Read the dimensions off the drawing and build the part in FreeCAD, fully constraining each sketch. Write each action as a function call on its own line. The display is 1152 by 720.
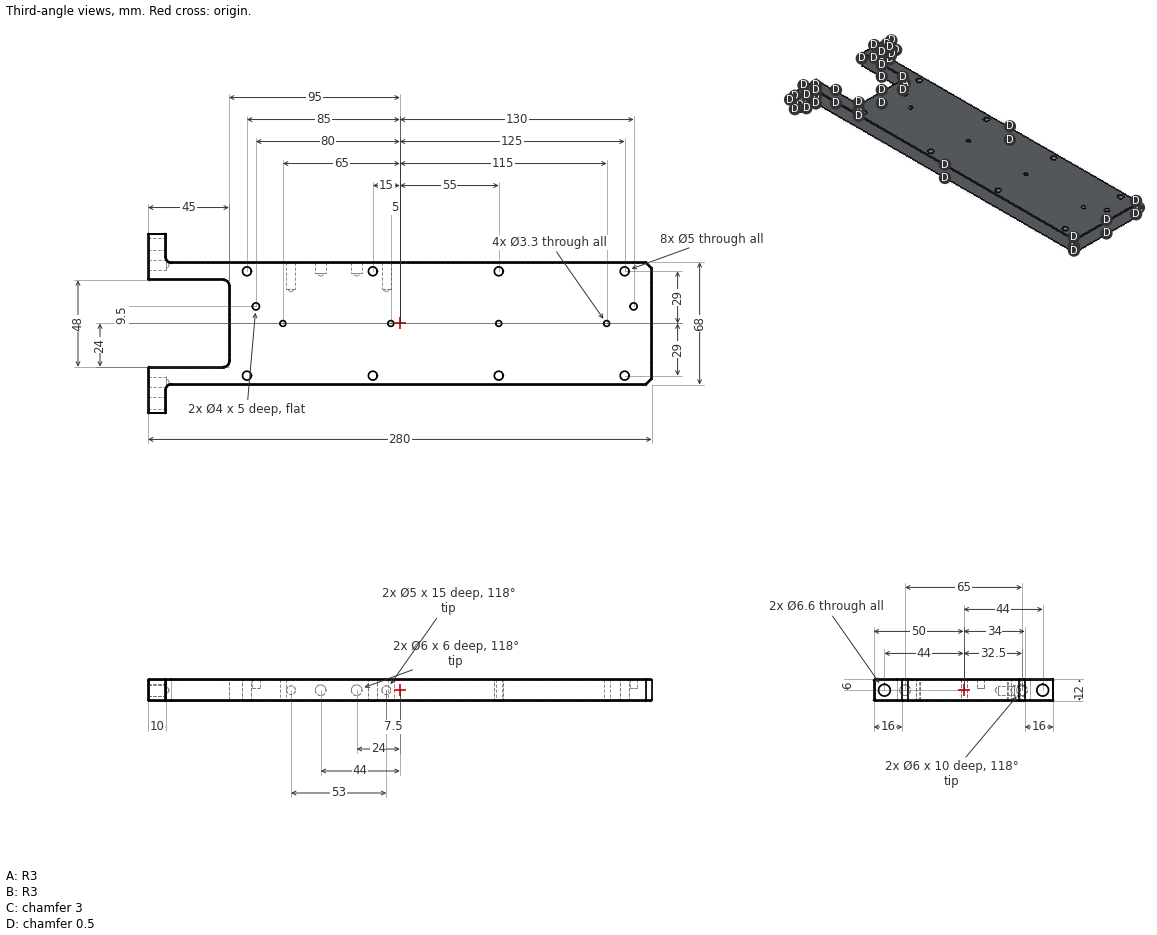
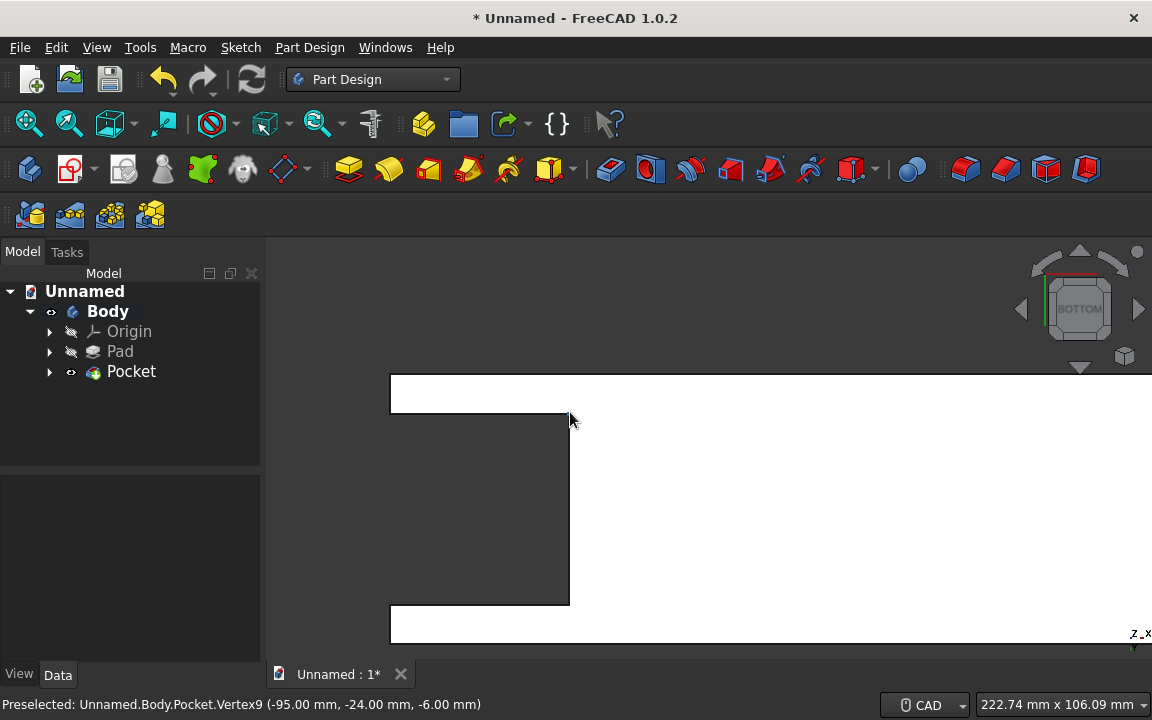
key(4)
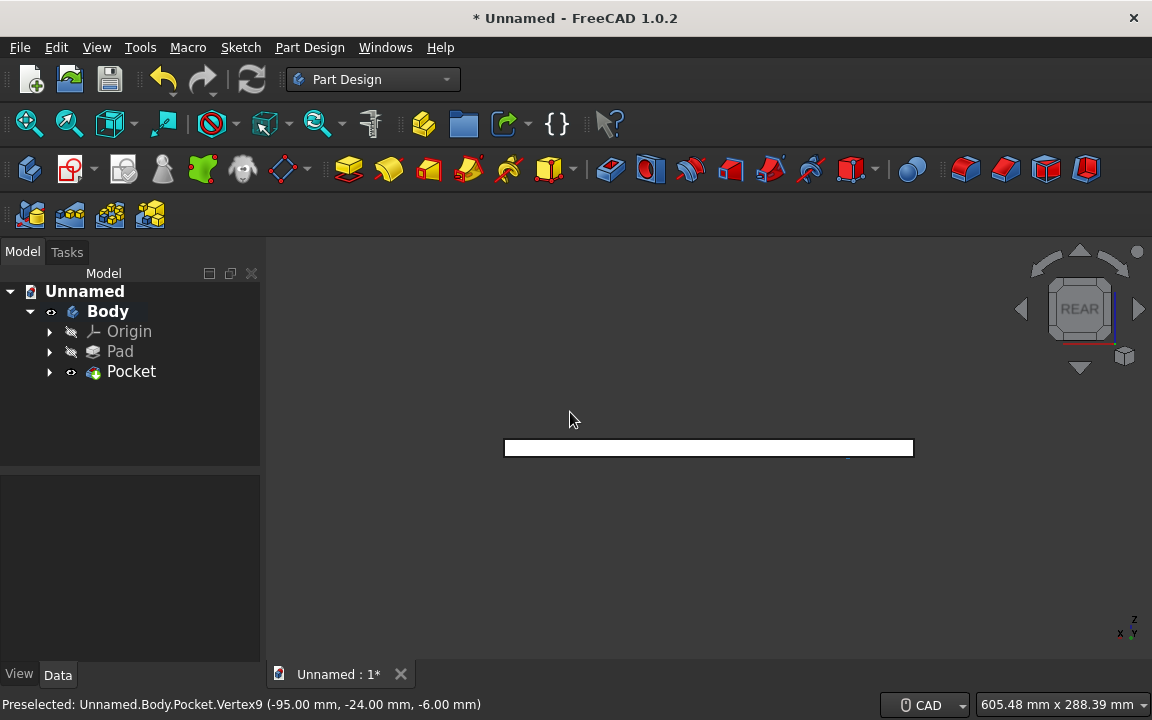
scroll(848, 447, up, 5)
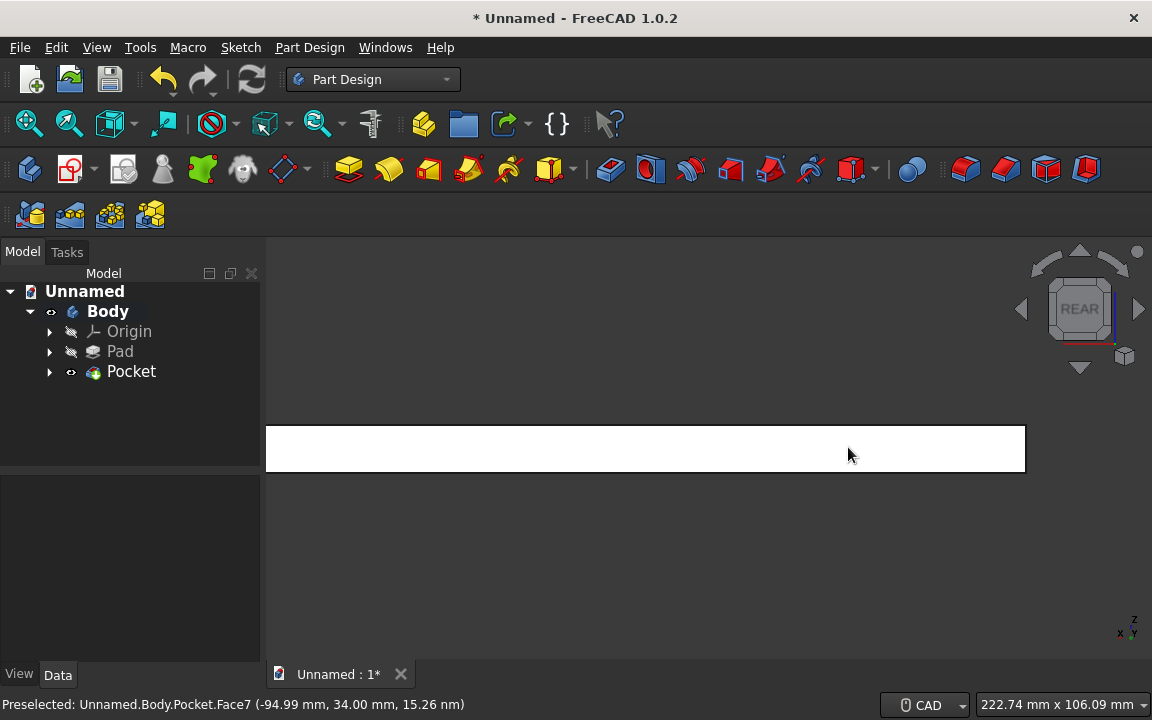
key(v)
key(f)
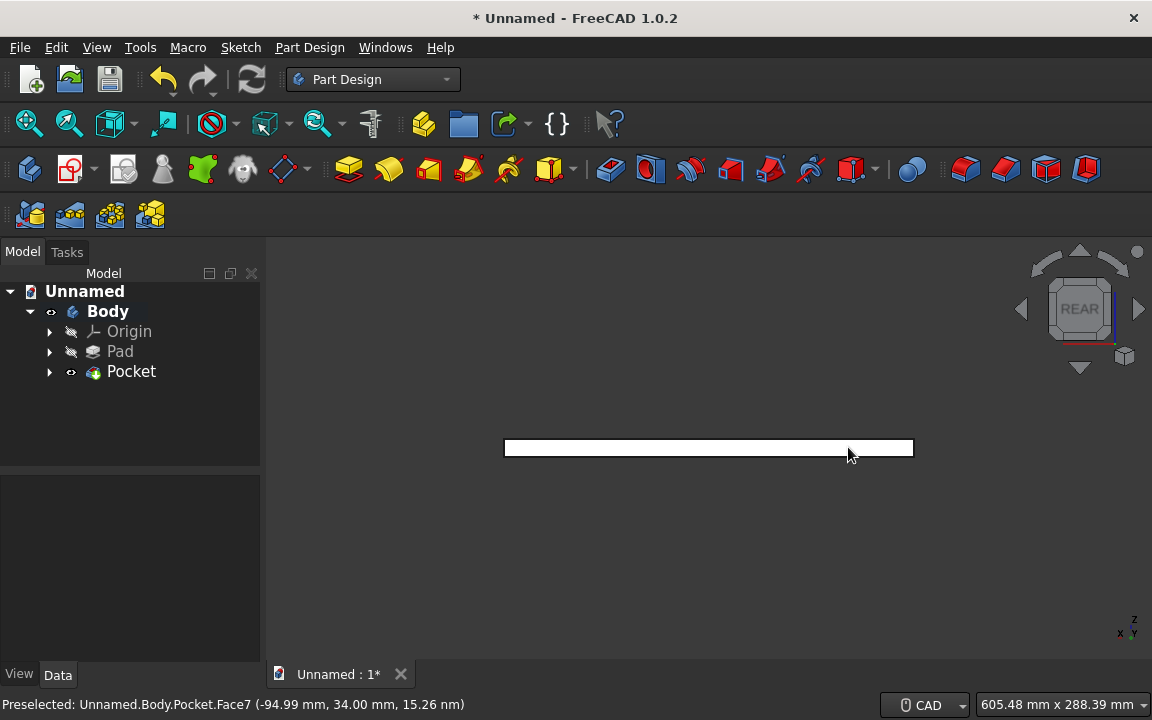
key(6)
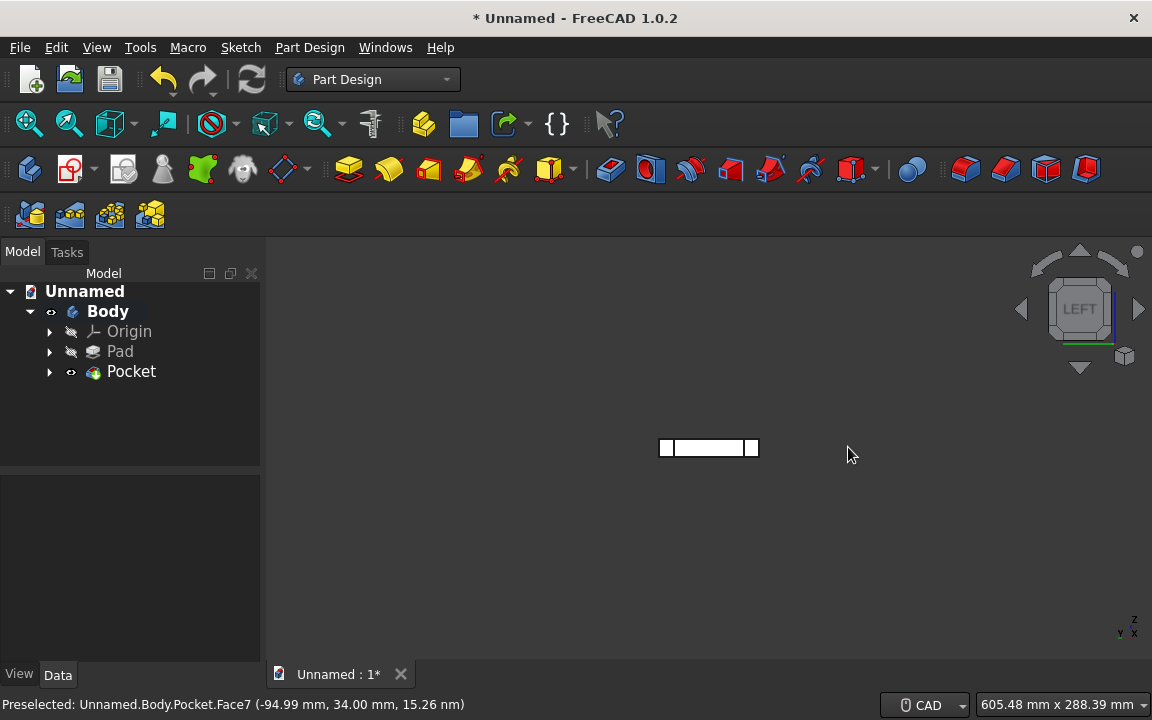
click(30, 124)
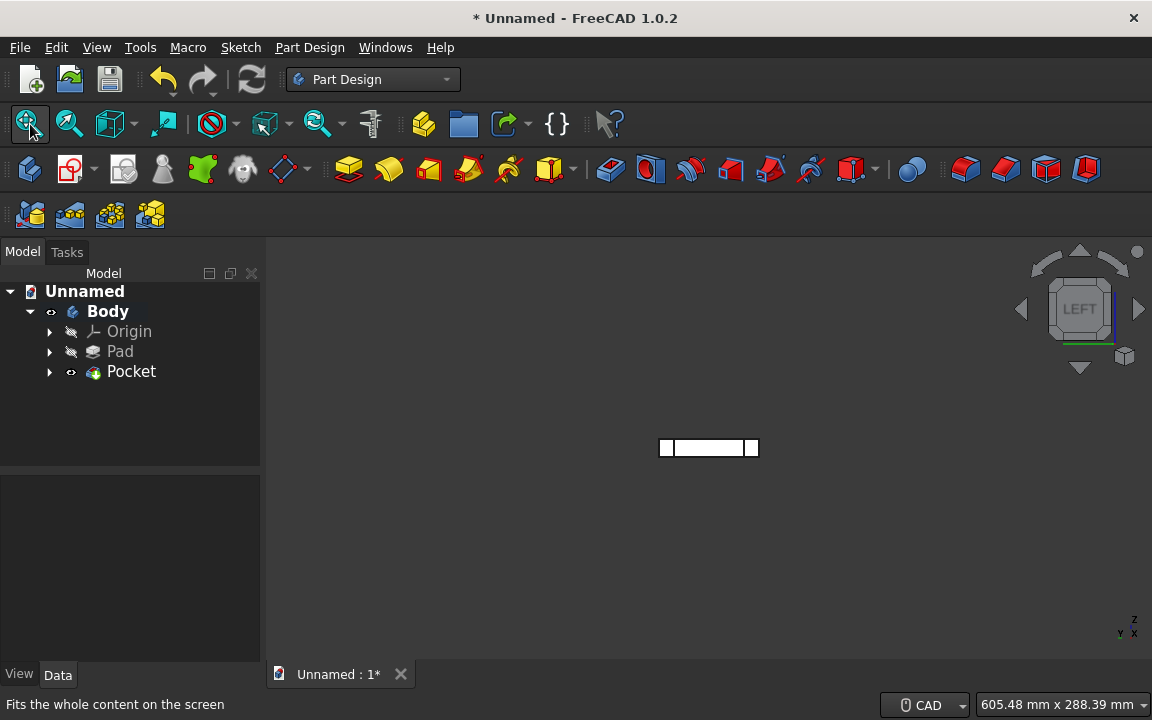
scroll(744, 447, up, 5)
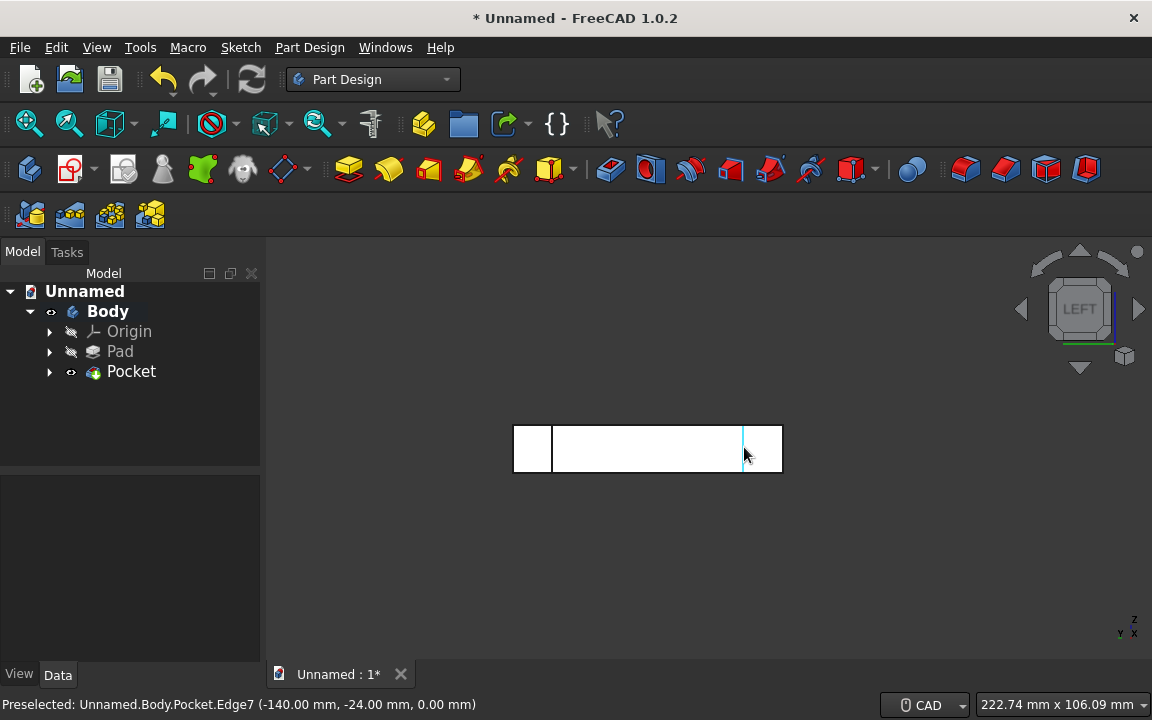
click(30, 124)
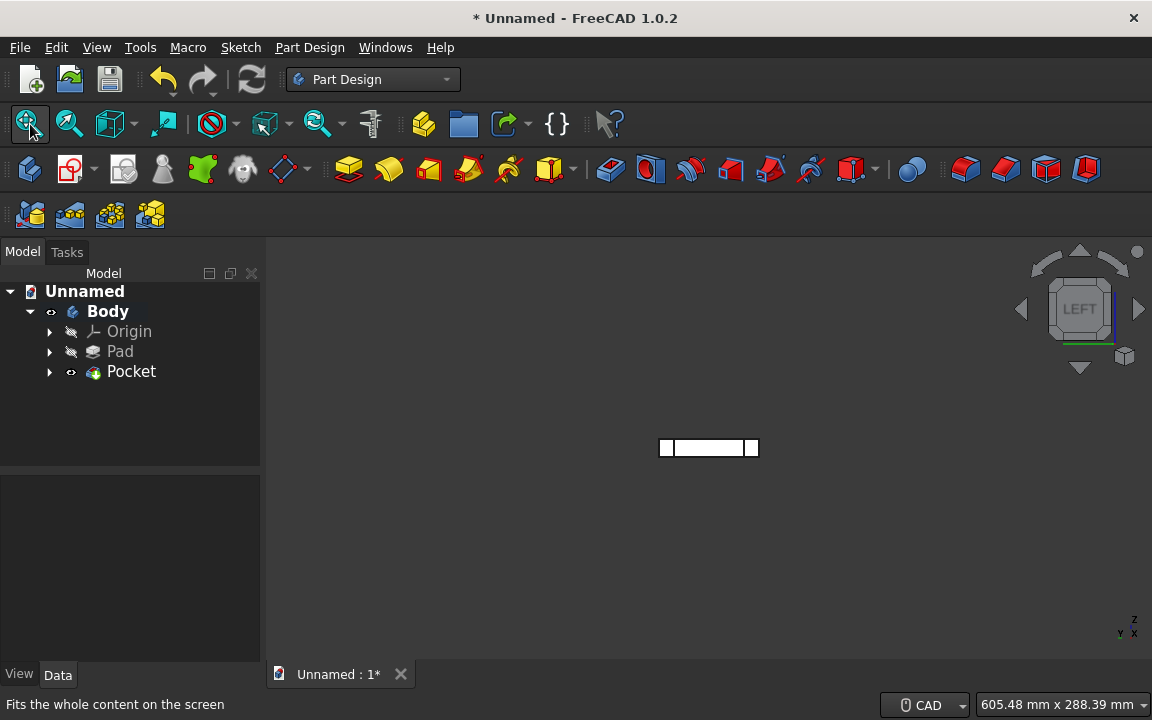
key(v)
key(3)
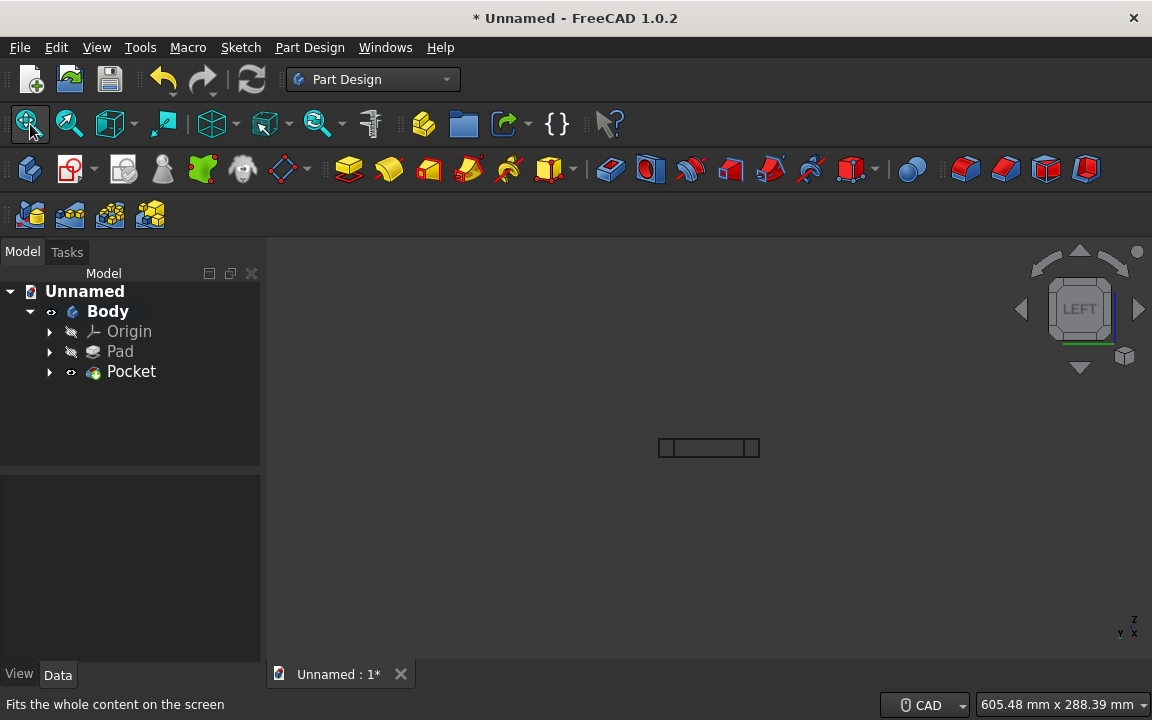
key(0)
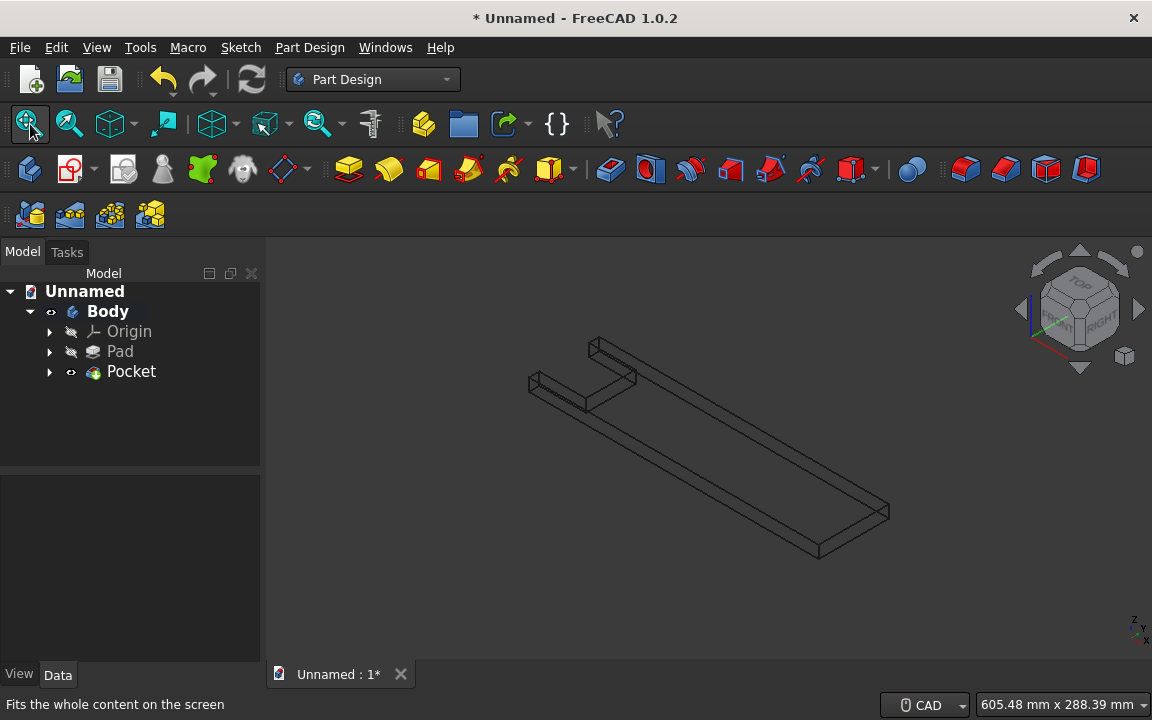
click(636, 376)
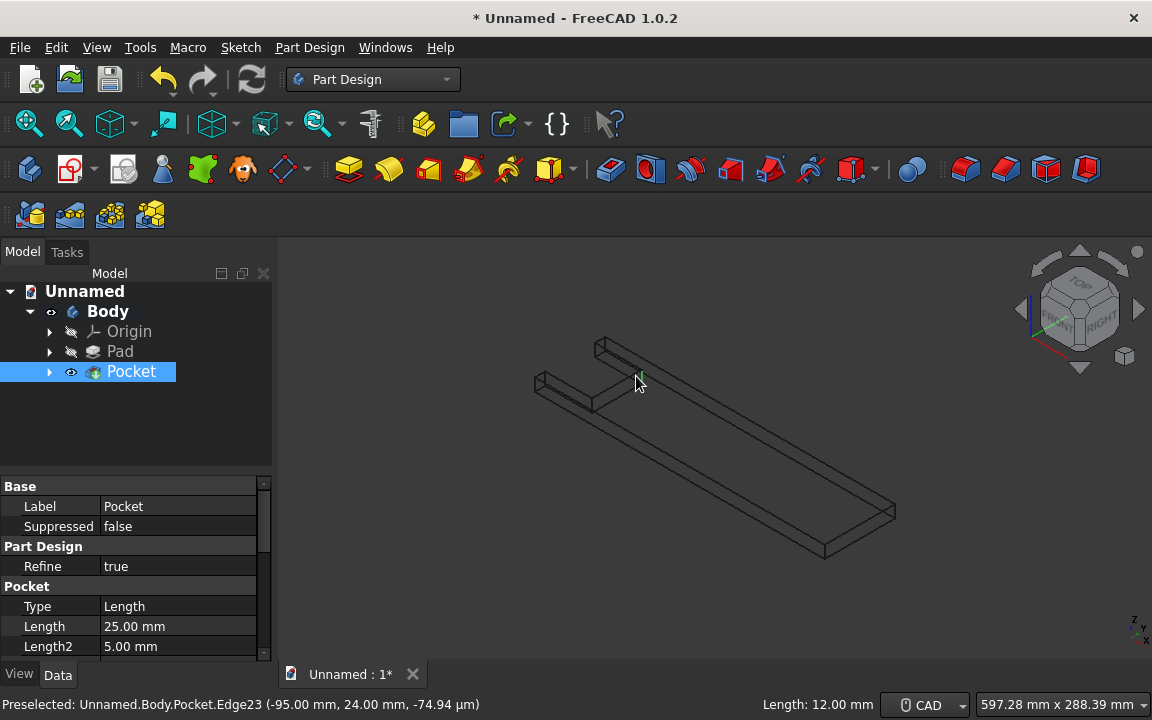
scroll(592, 405, up, 6)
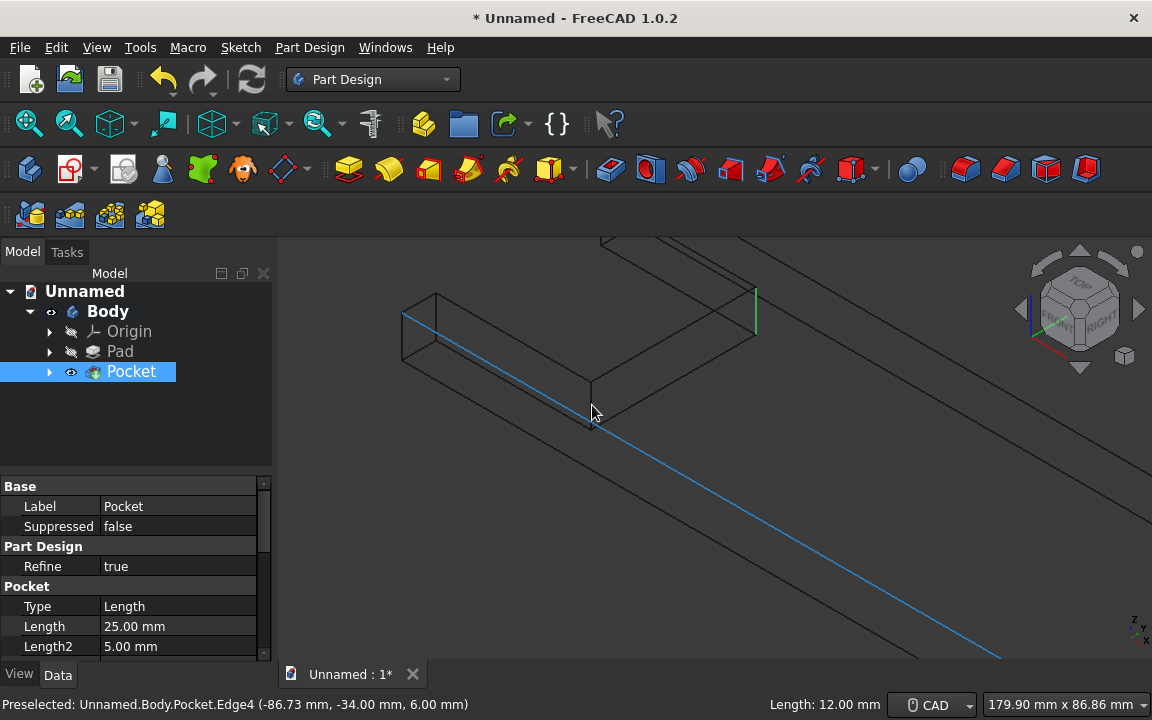
click(591, 405, ctrl)